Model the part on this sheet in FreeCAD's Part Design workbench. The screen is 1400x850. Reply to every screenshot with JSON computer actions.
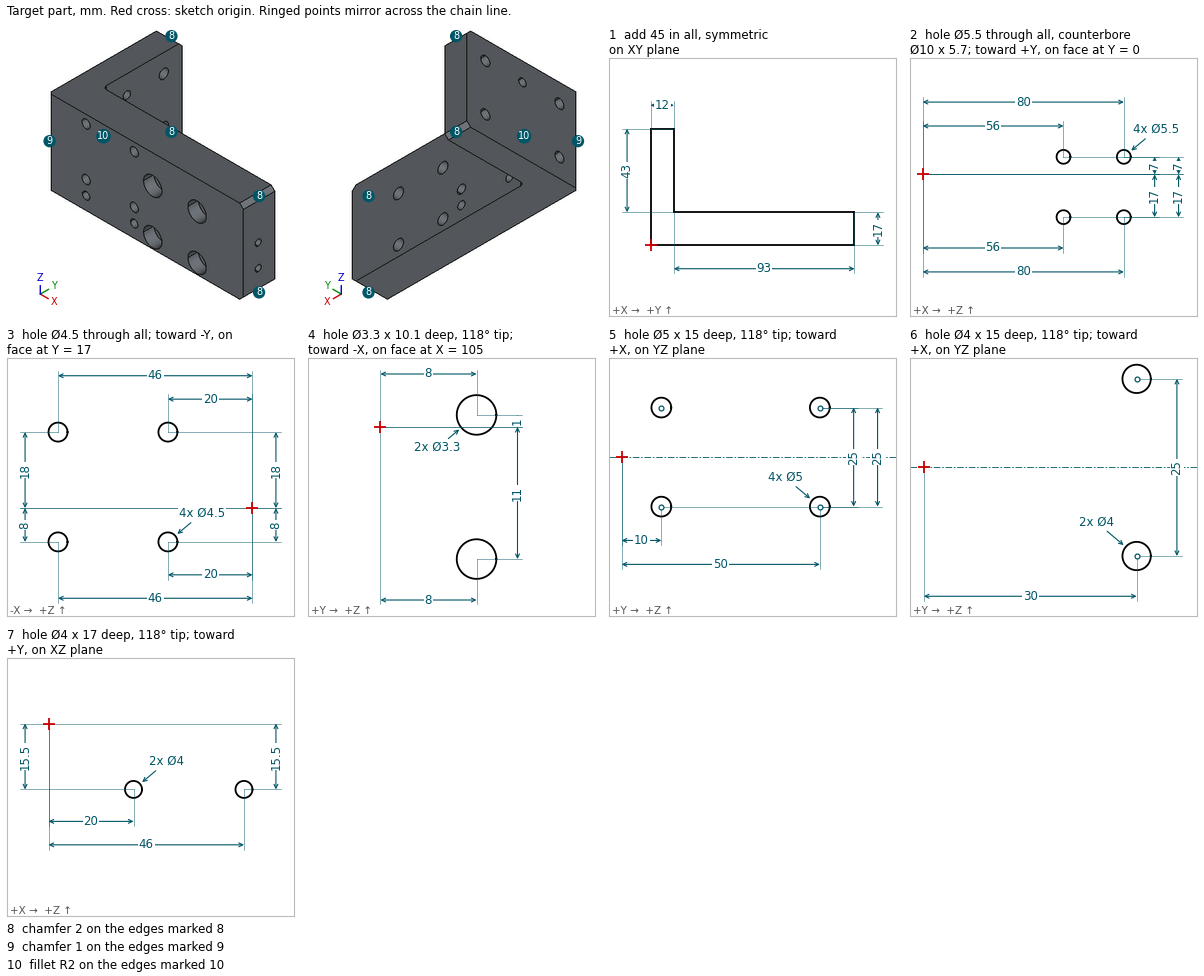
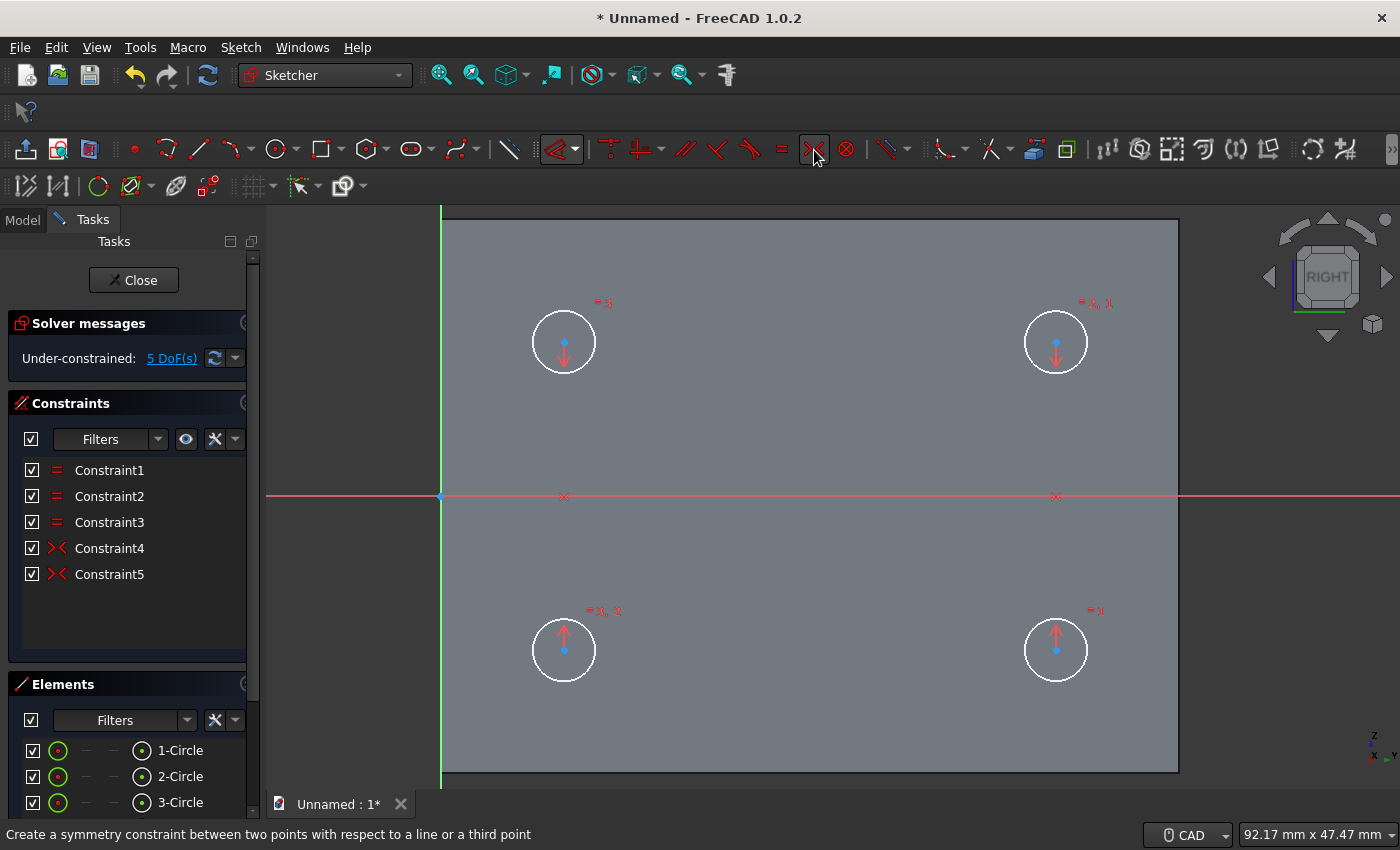
{"action": "left_click", "coordinate": [1078, 628]}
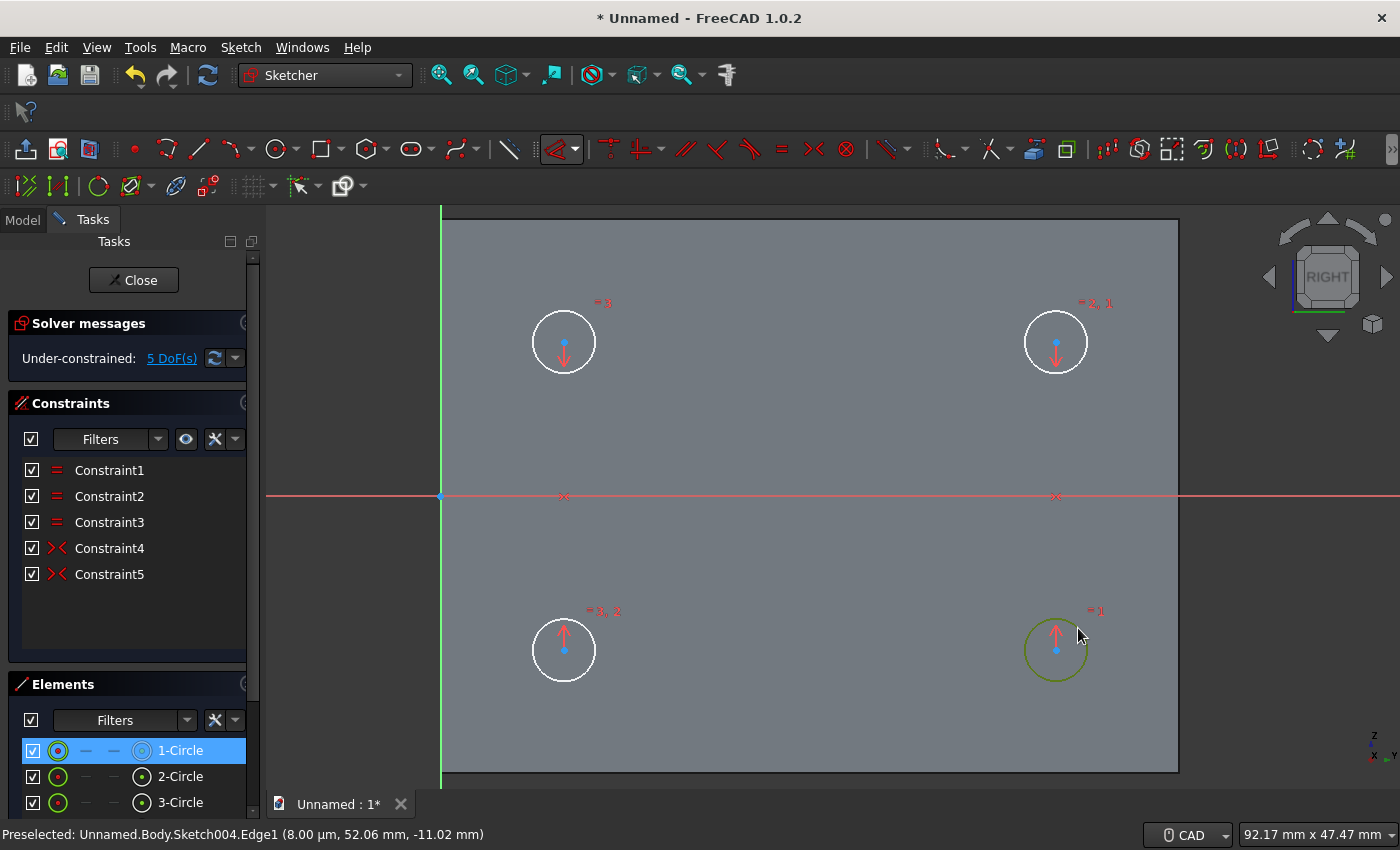
{"action": "key", "text": "k o"}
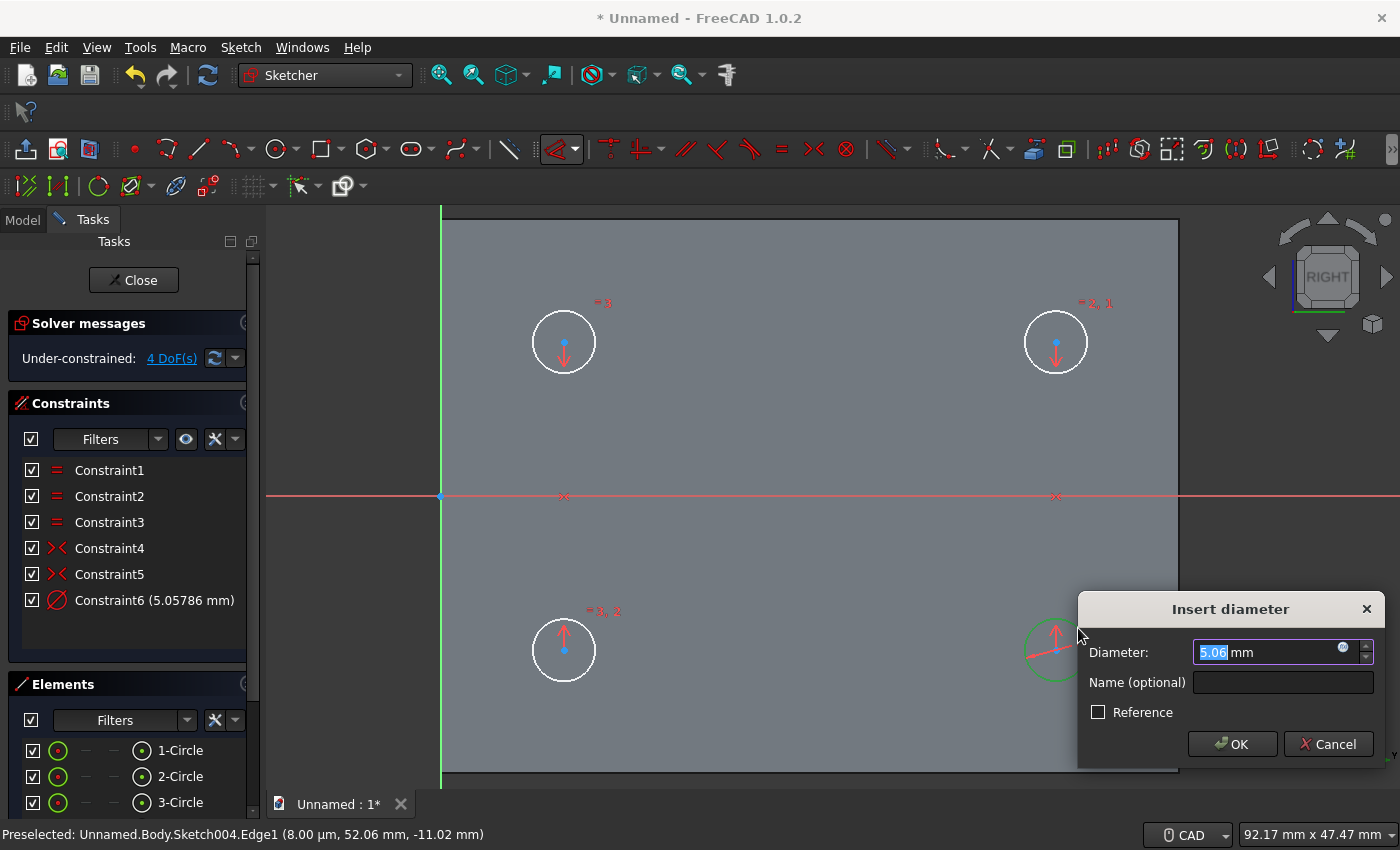
{"action": "type", "text": "5"}
{"action": "key", "text": "Return"}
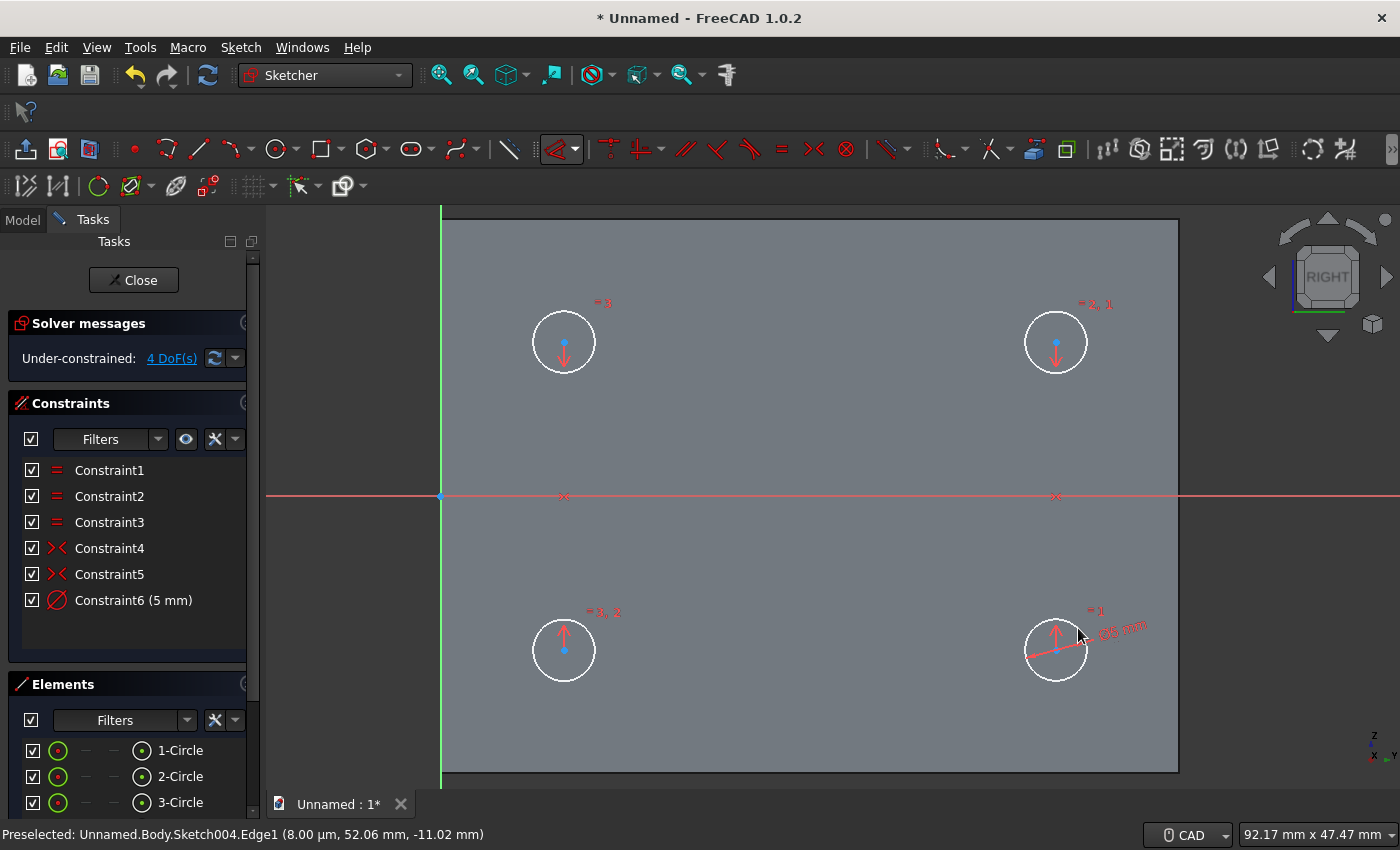
{"action": "left_click", "coordinate": [1056, 650]}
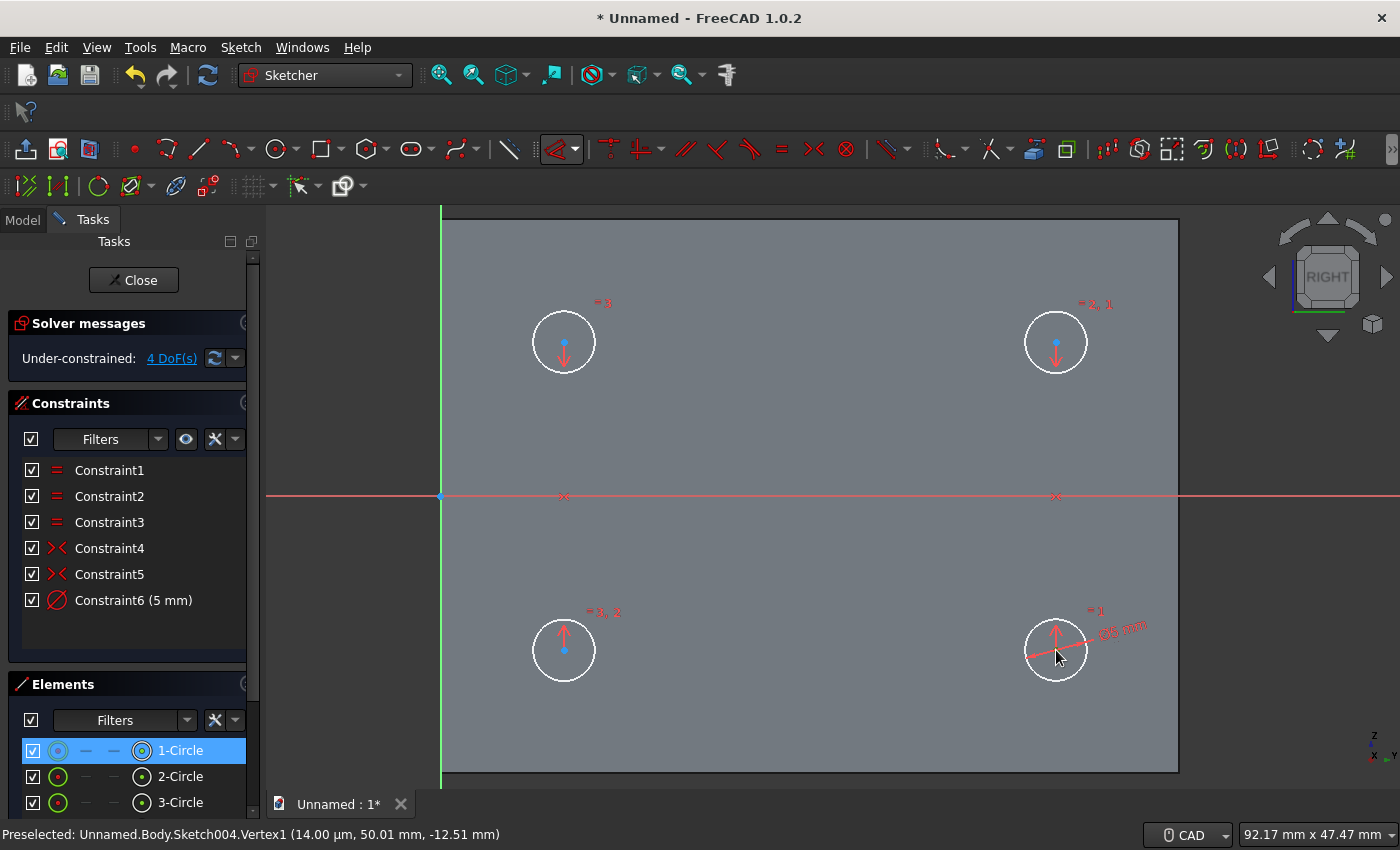
{"action": "key", "text": "l"}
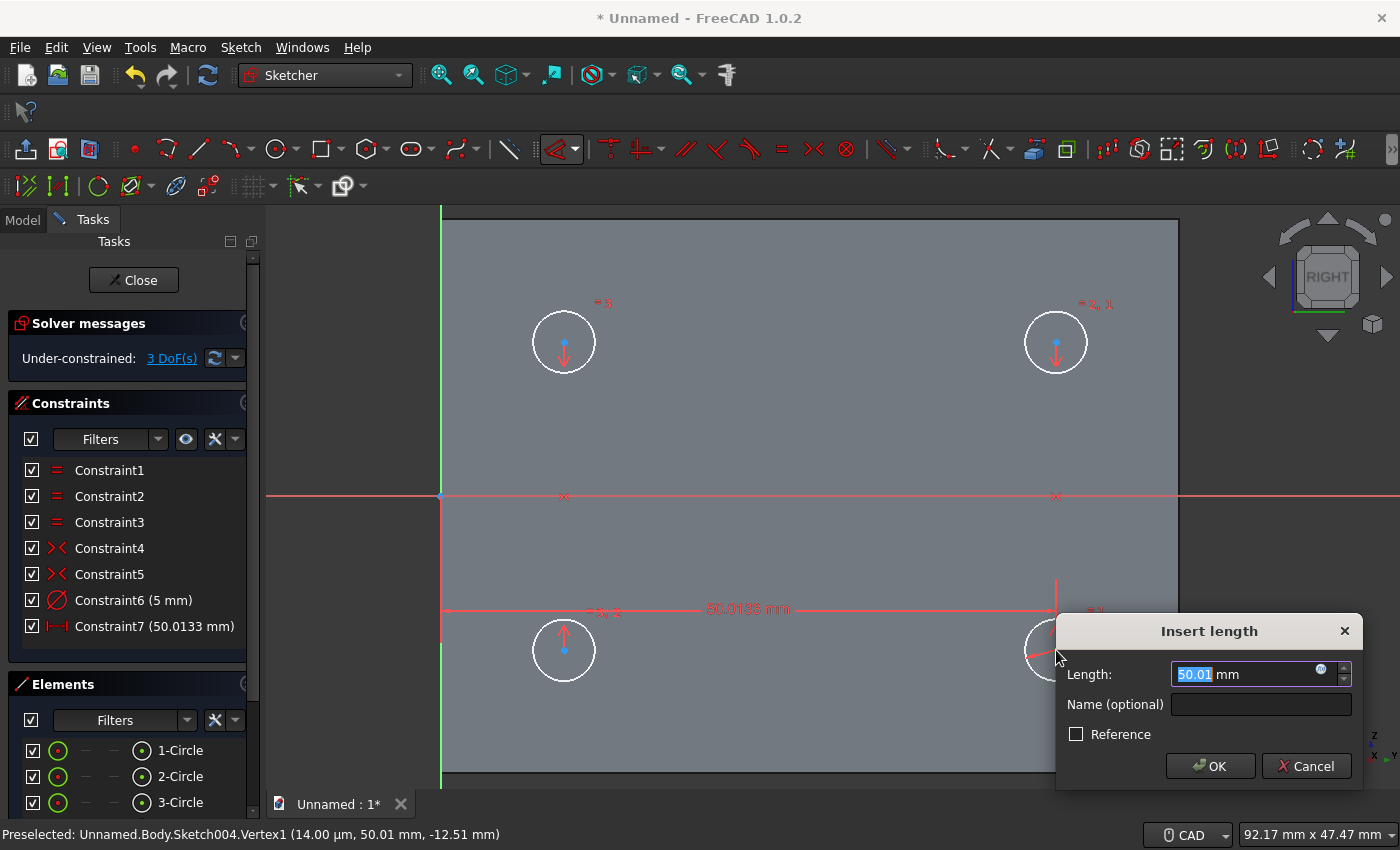
{"action": "type", "text": "50"}
{"action": "key", "text": "Return"}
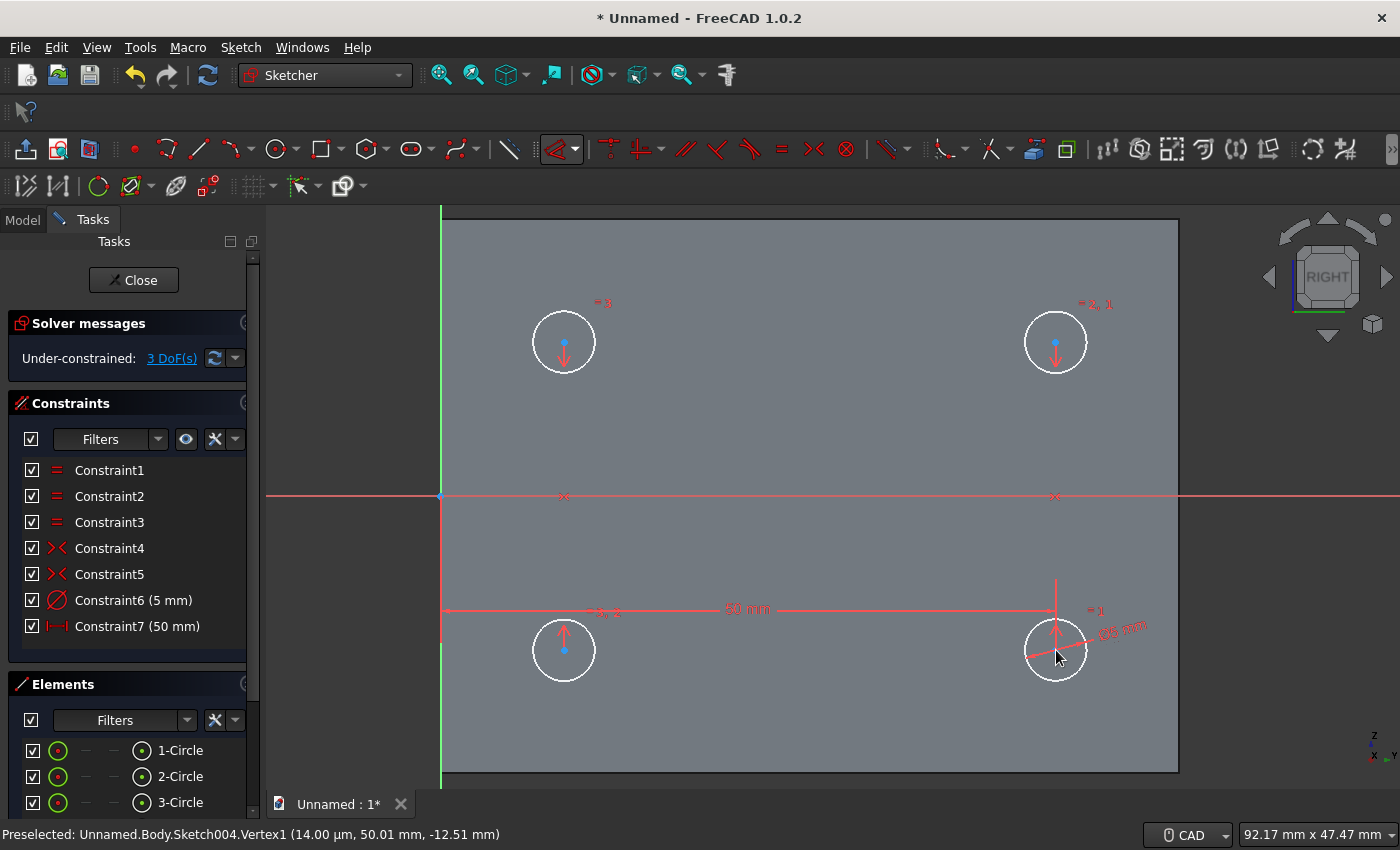
{"action": "left_click", "coordinate": [564, 650]}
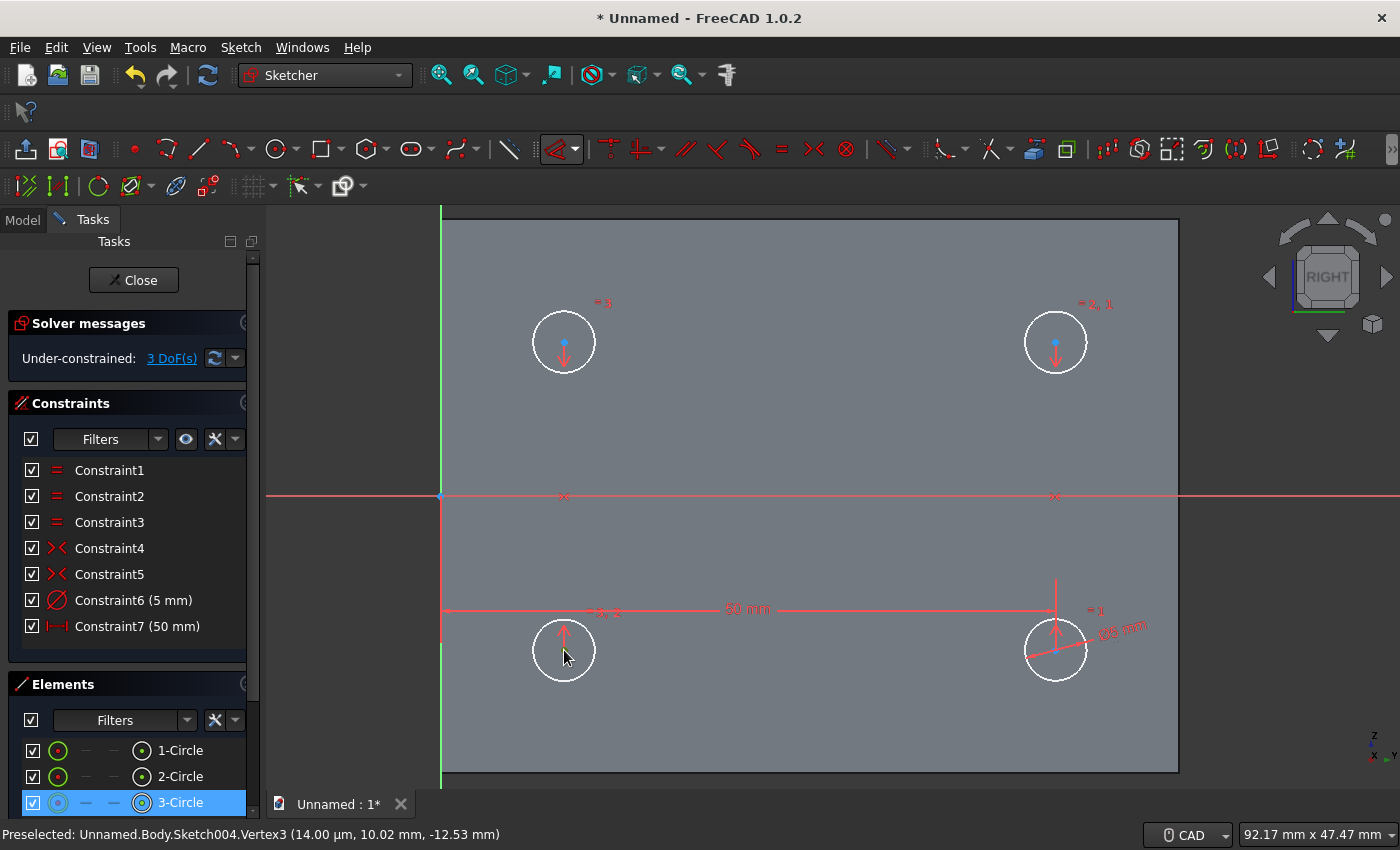
{"action": "key", "text": "l"}